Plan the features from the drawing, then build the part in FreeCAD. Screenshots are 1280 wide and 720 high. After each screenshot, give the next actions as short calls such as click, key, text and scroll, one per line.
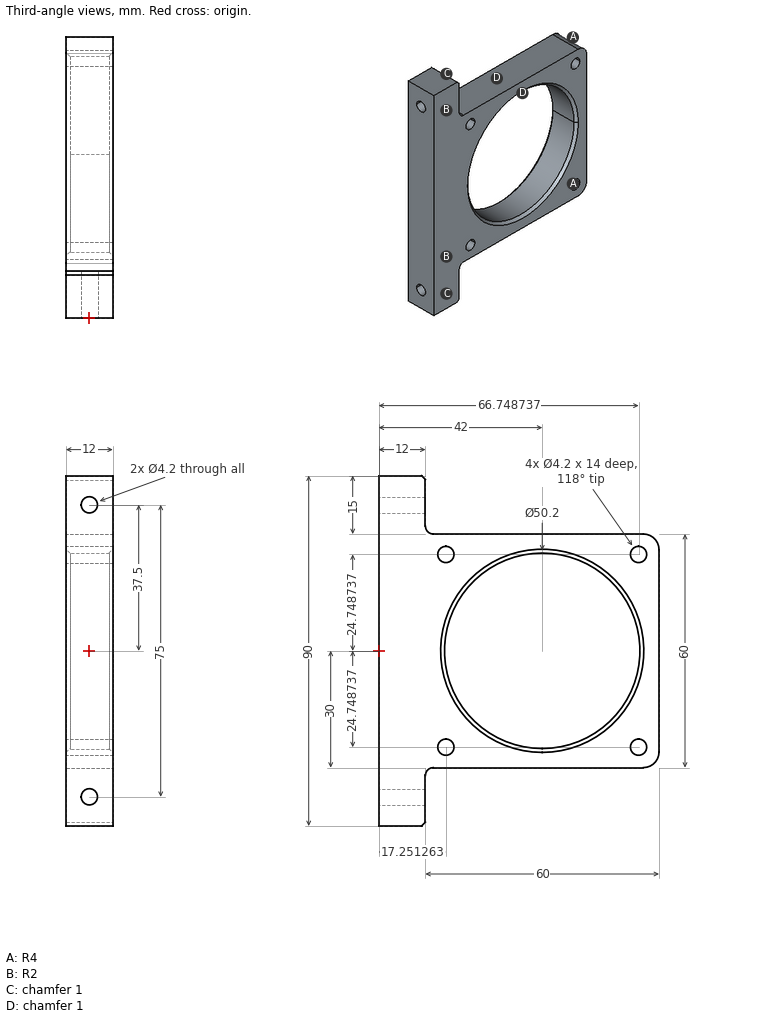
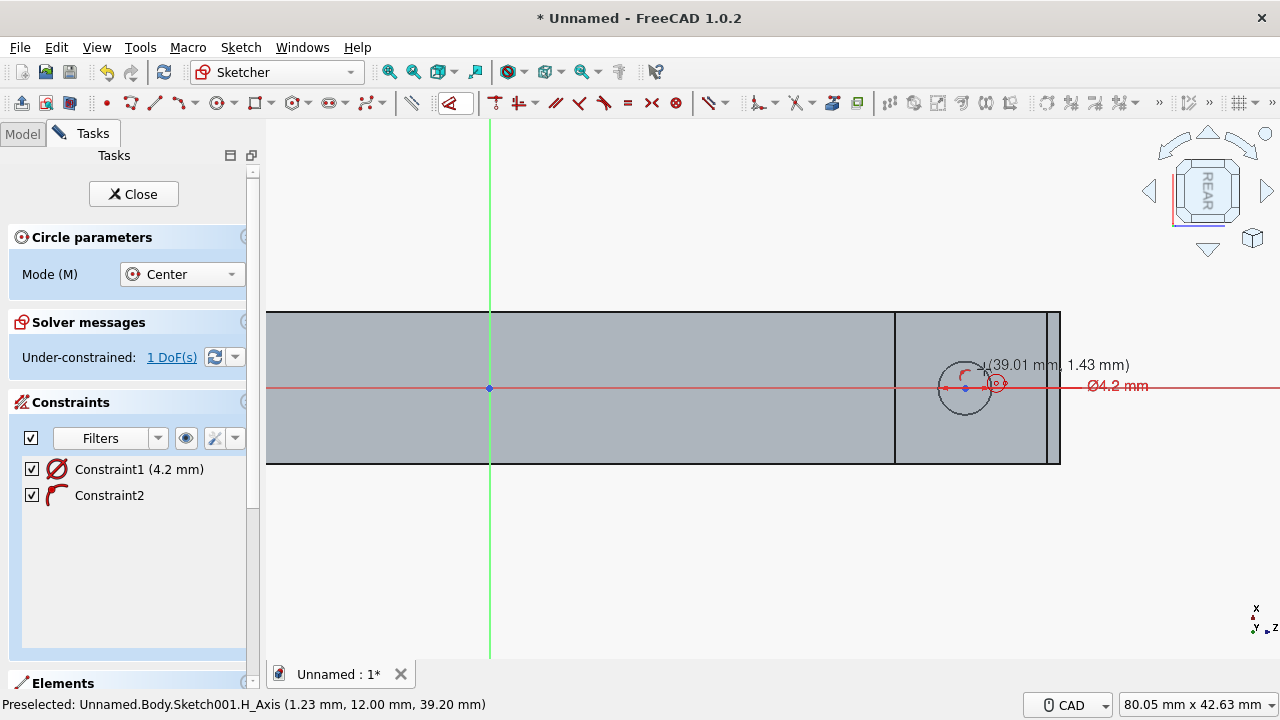
scroll(966, 390, down, 3)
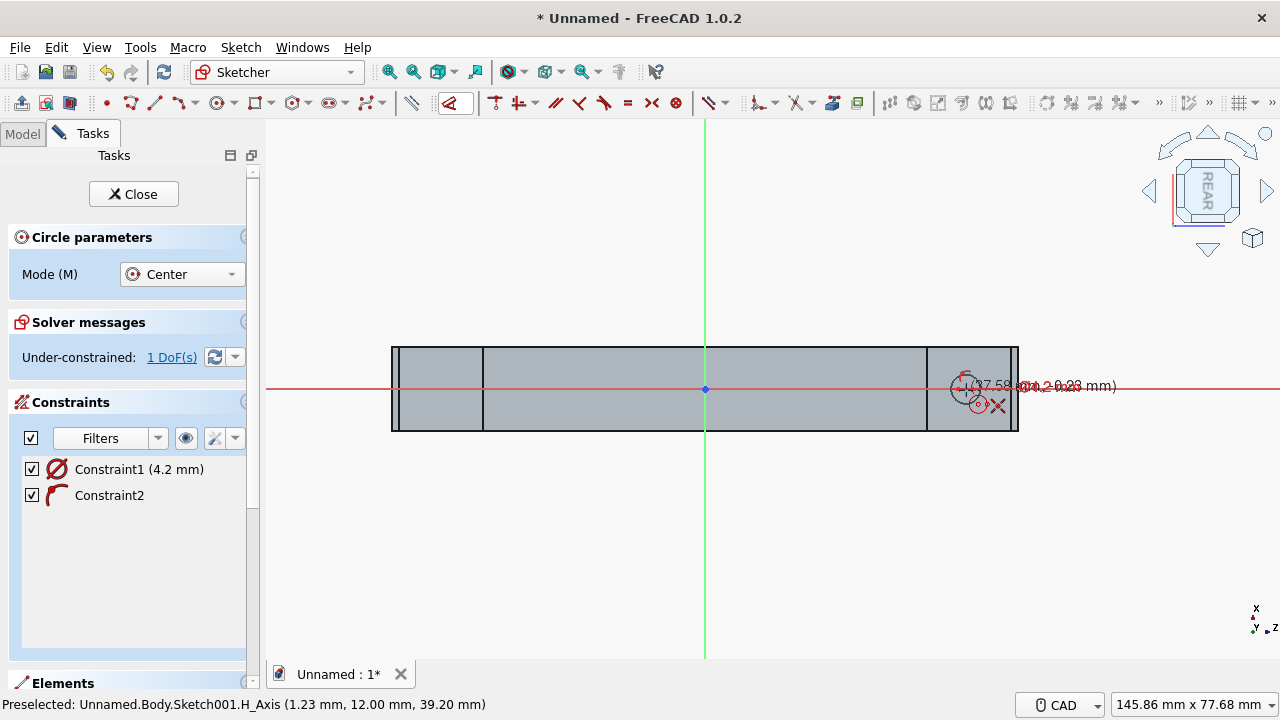
scroll(444, 389, up, 3)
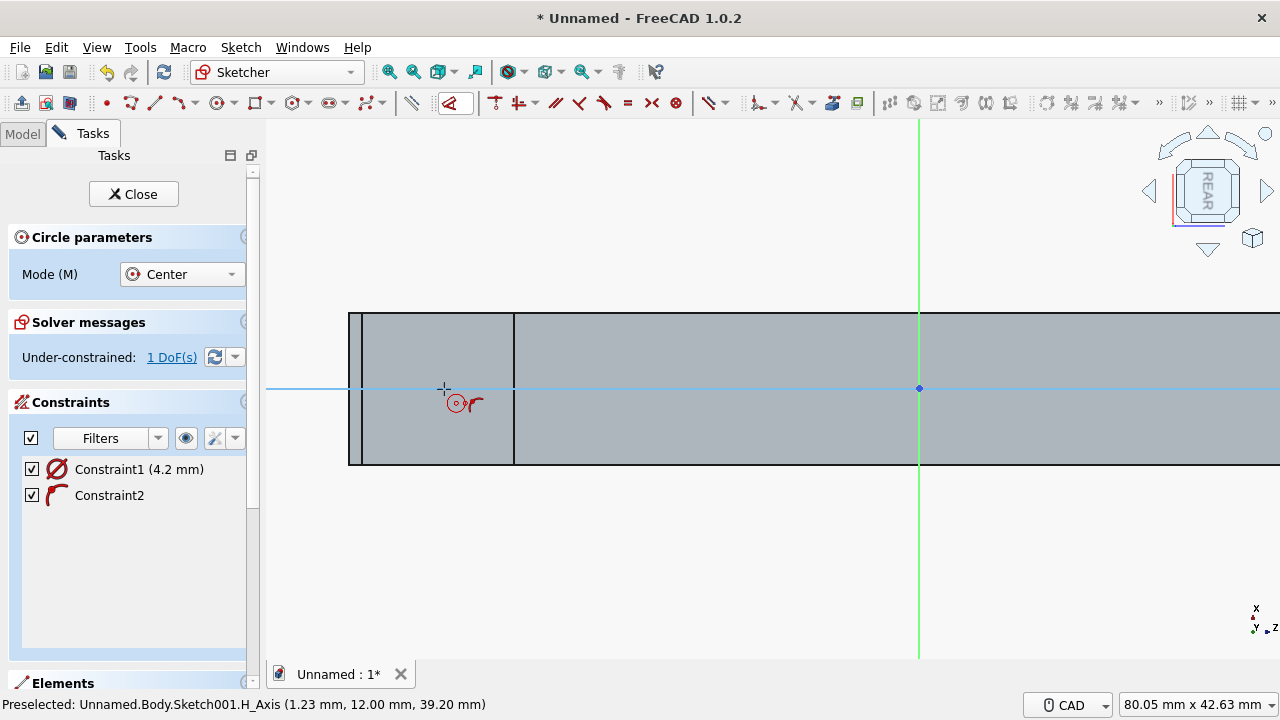
click(444, 389)
move(463, 370)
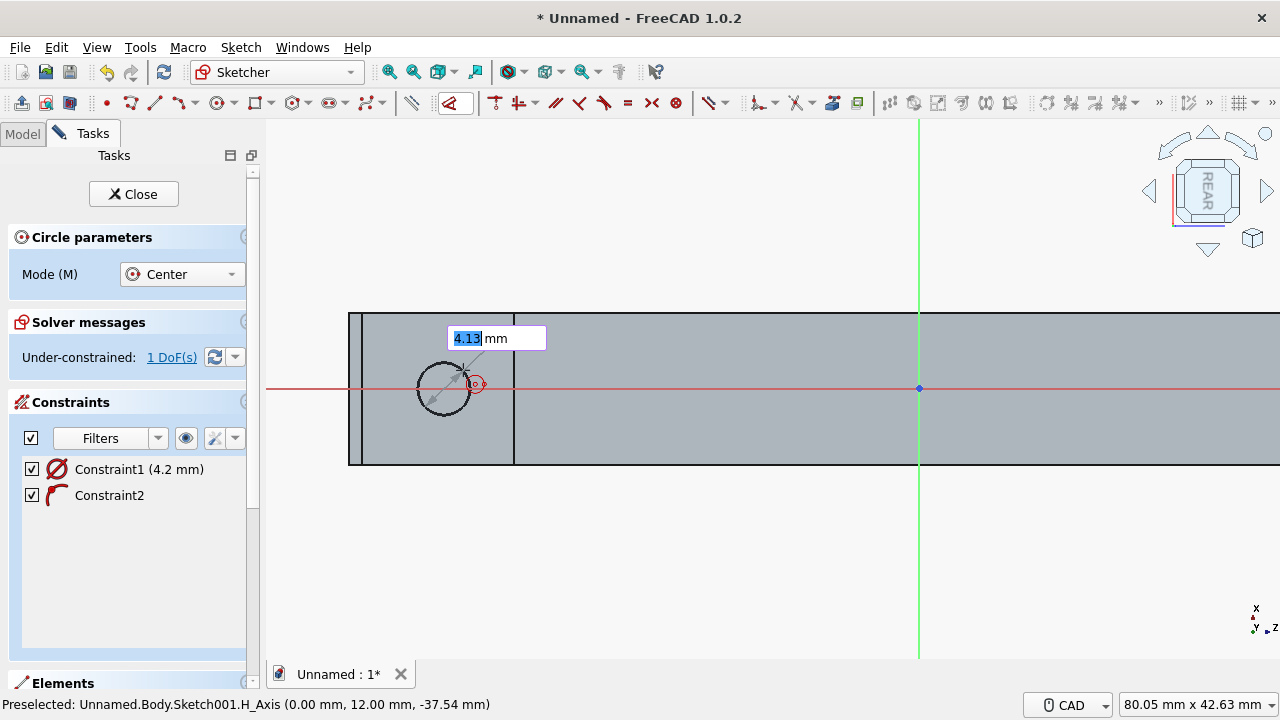
text(4.2)
key(Return)
key(Escape)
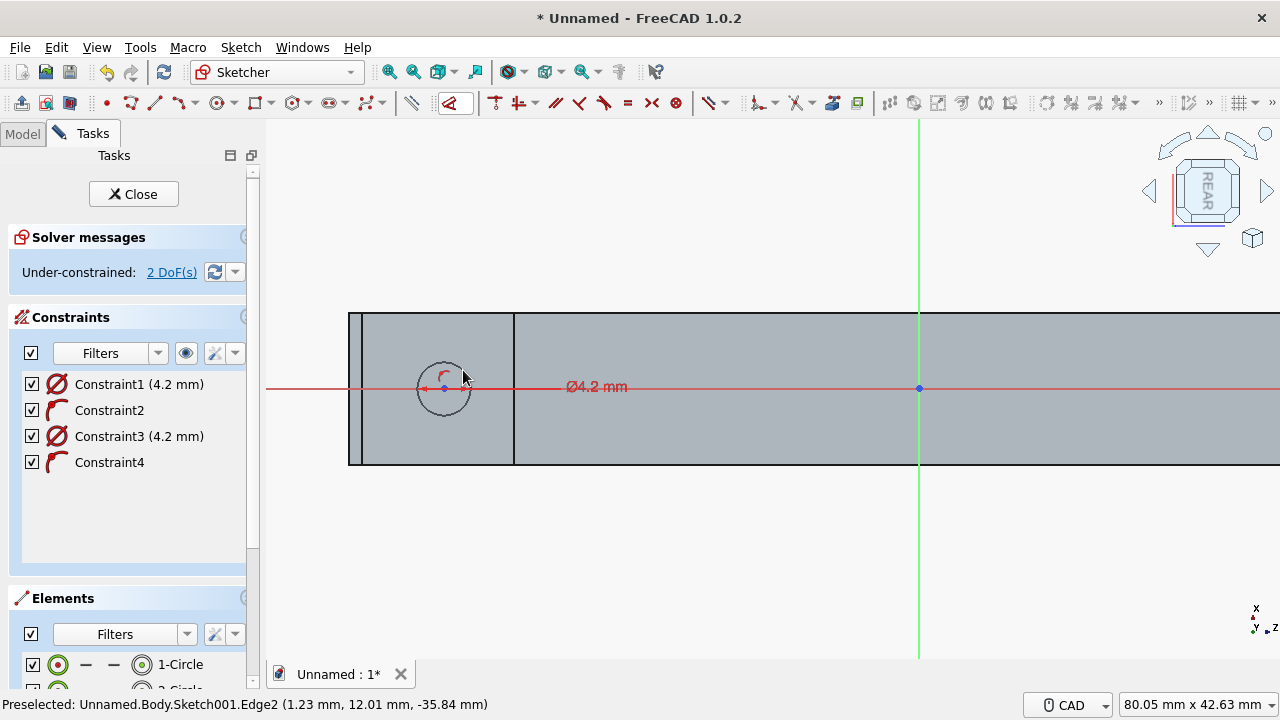
scroll(443, 389, down, 3)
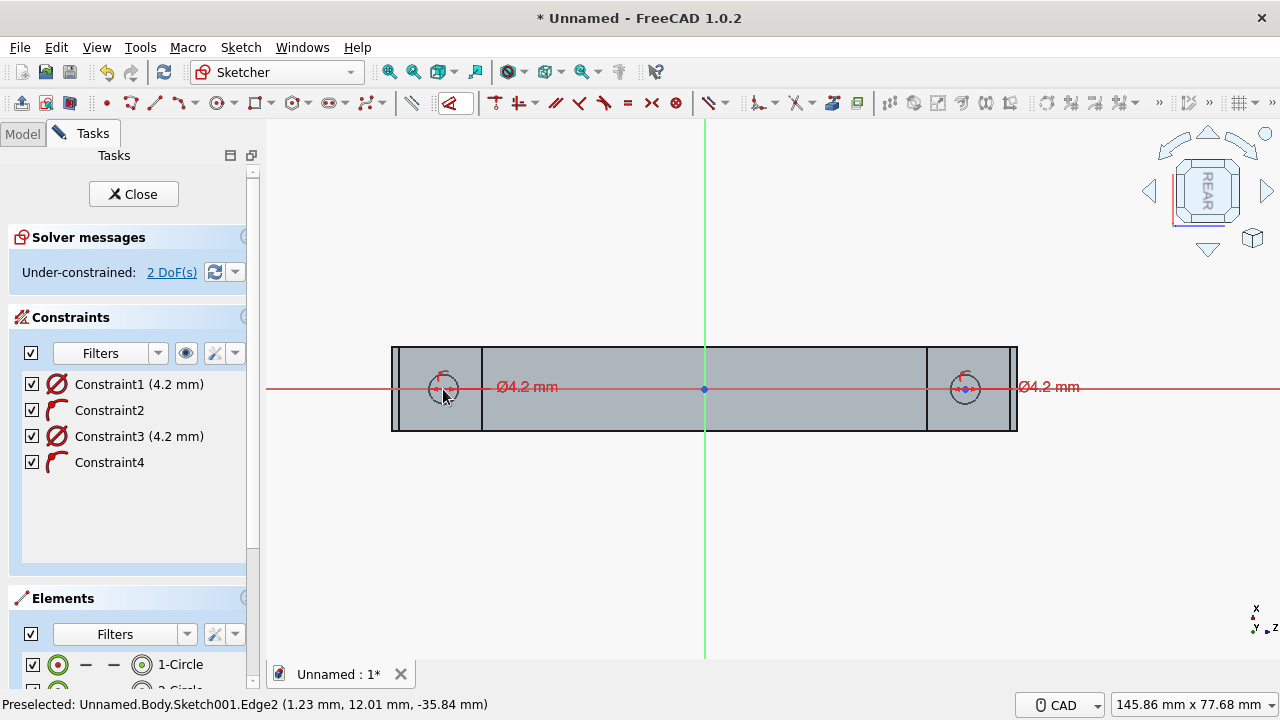
click(965, 389)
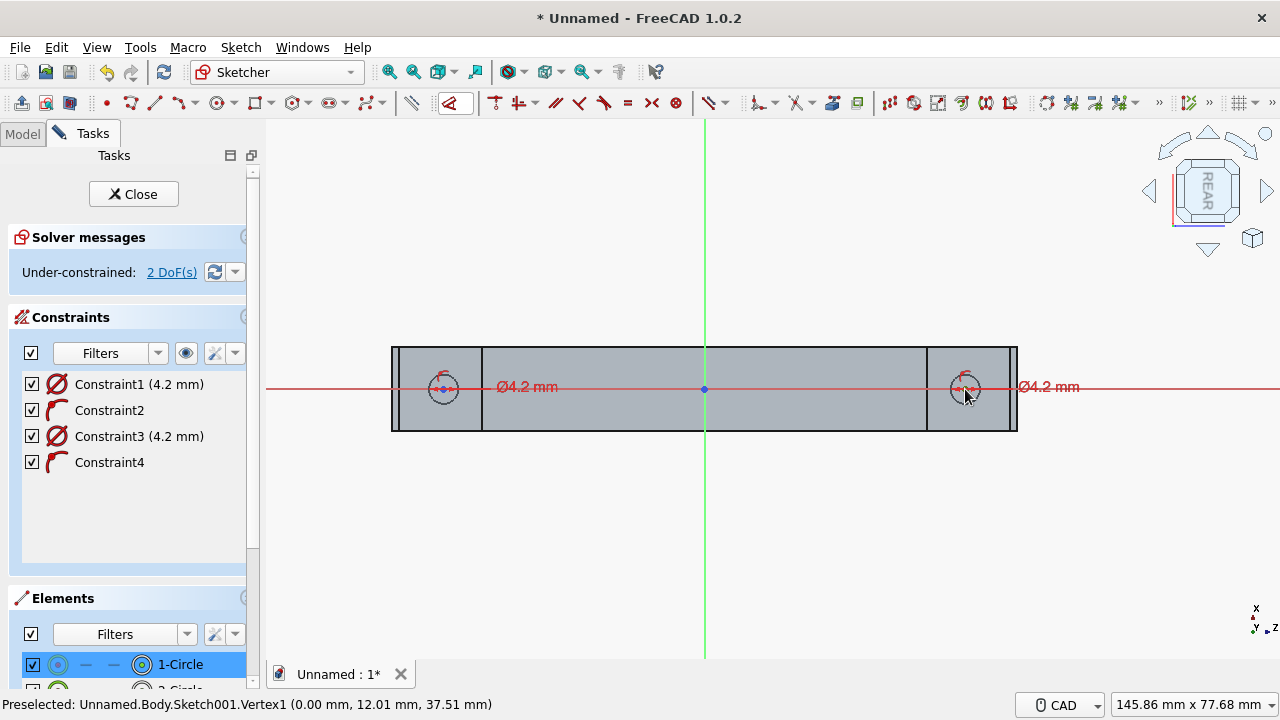
click(444, 389)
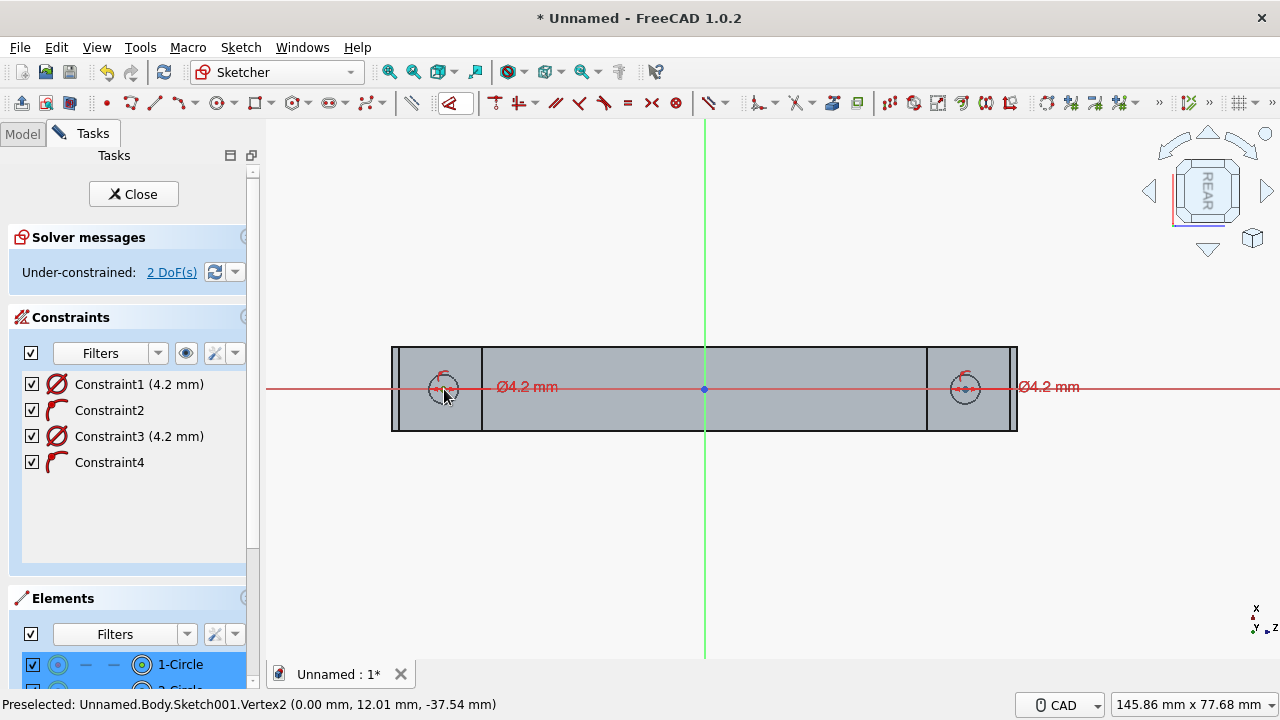
click(468, 104)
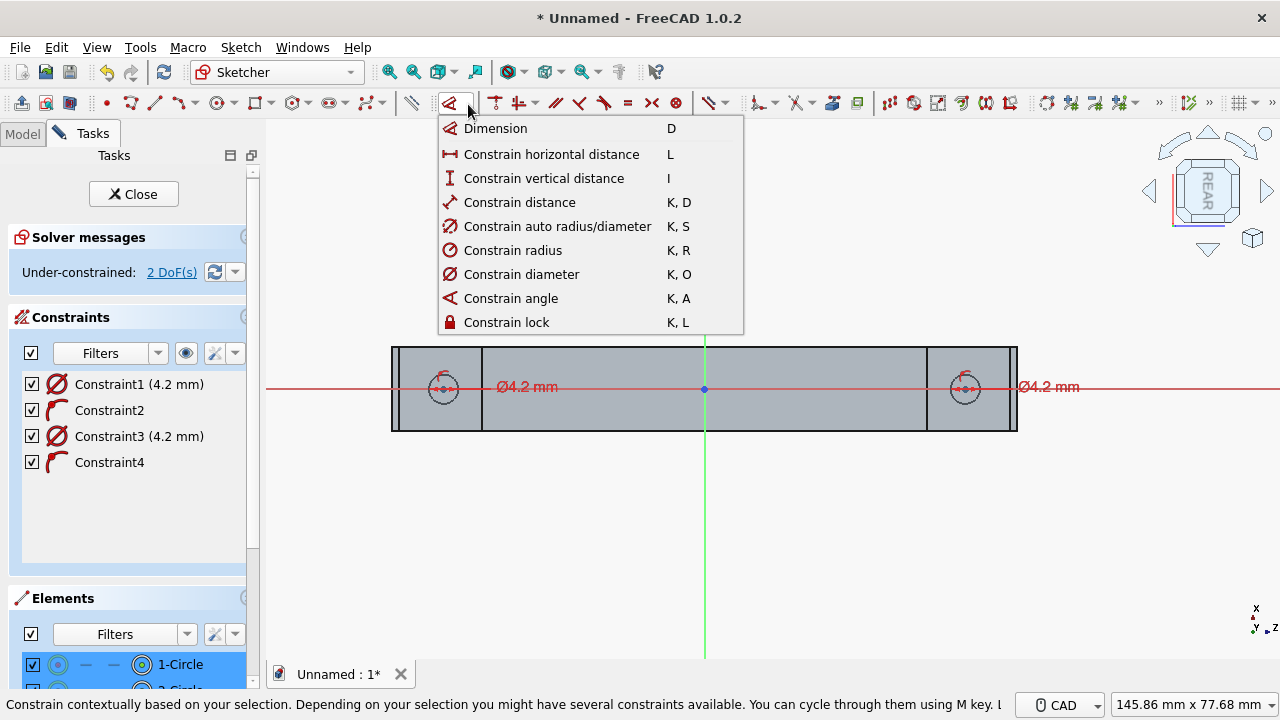
click(591, 154)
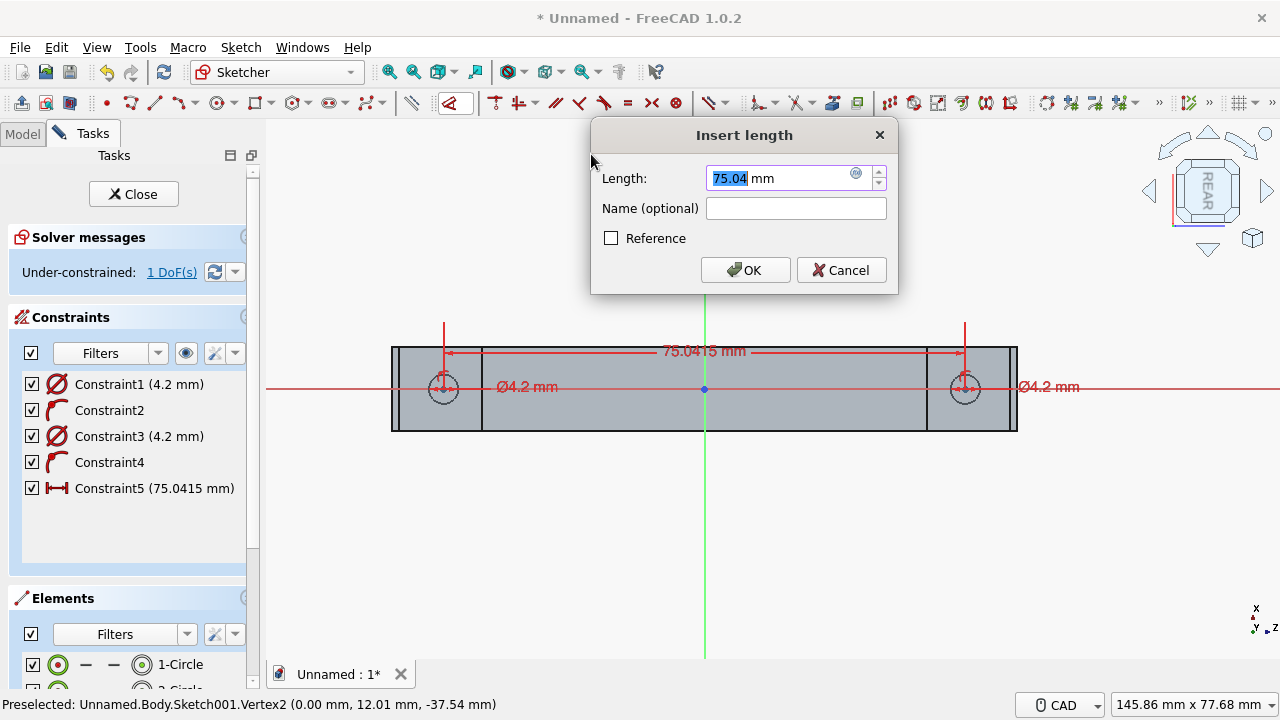
text(75)
key(Return)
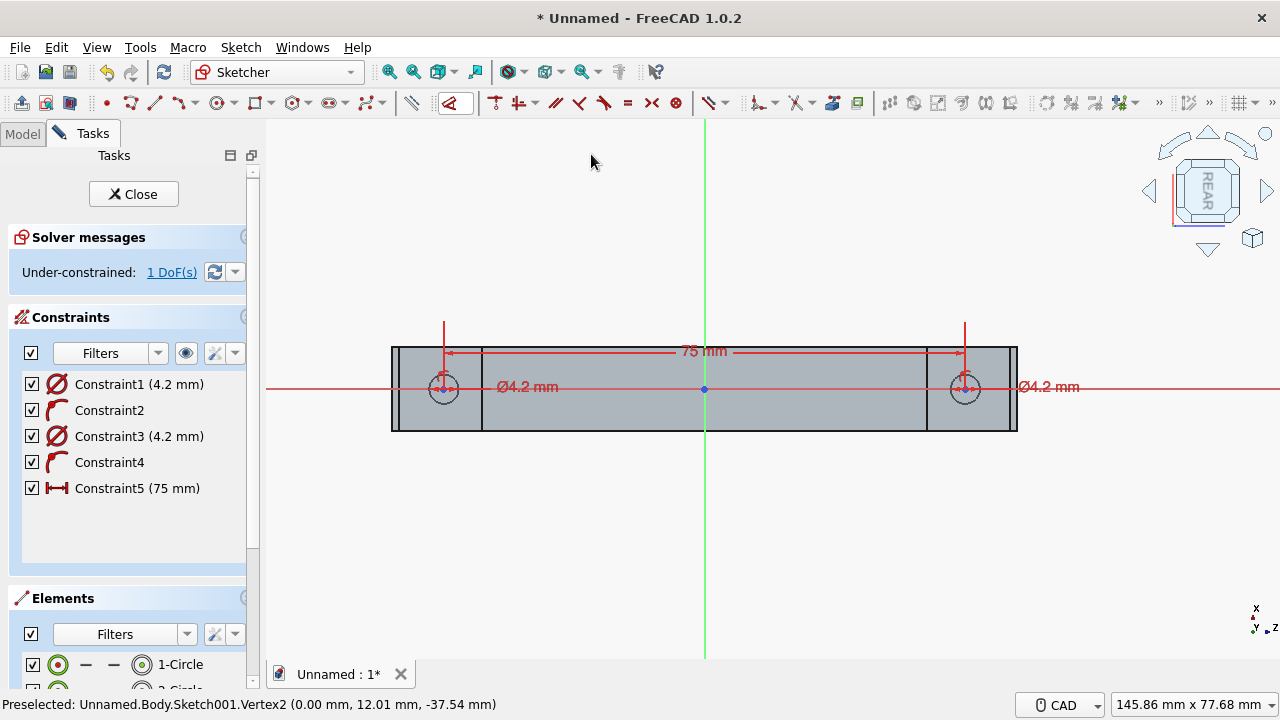
click(965, 389)